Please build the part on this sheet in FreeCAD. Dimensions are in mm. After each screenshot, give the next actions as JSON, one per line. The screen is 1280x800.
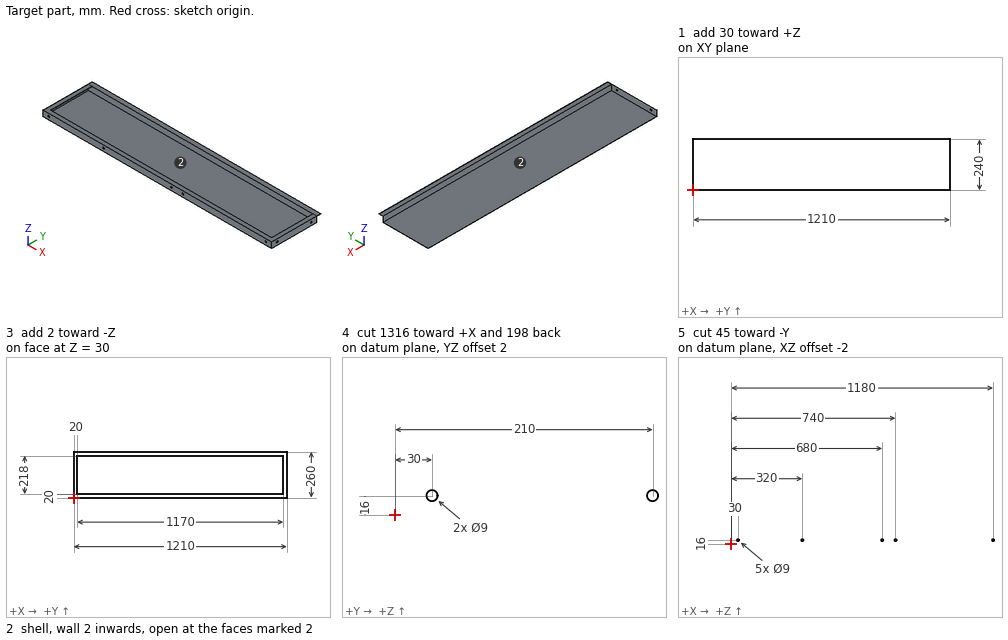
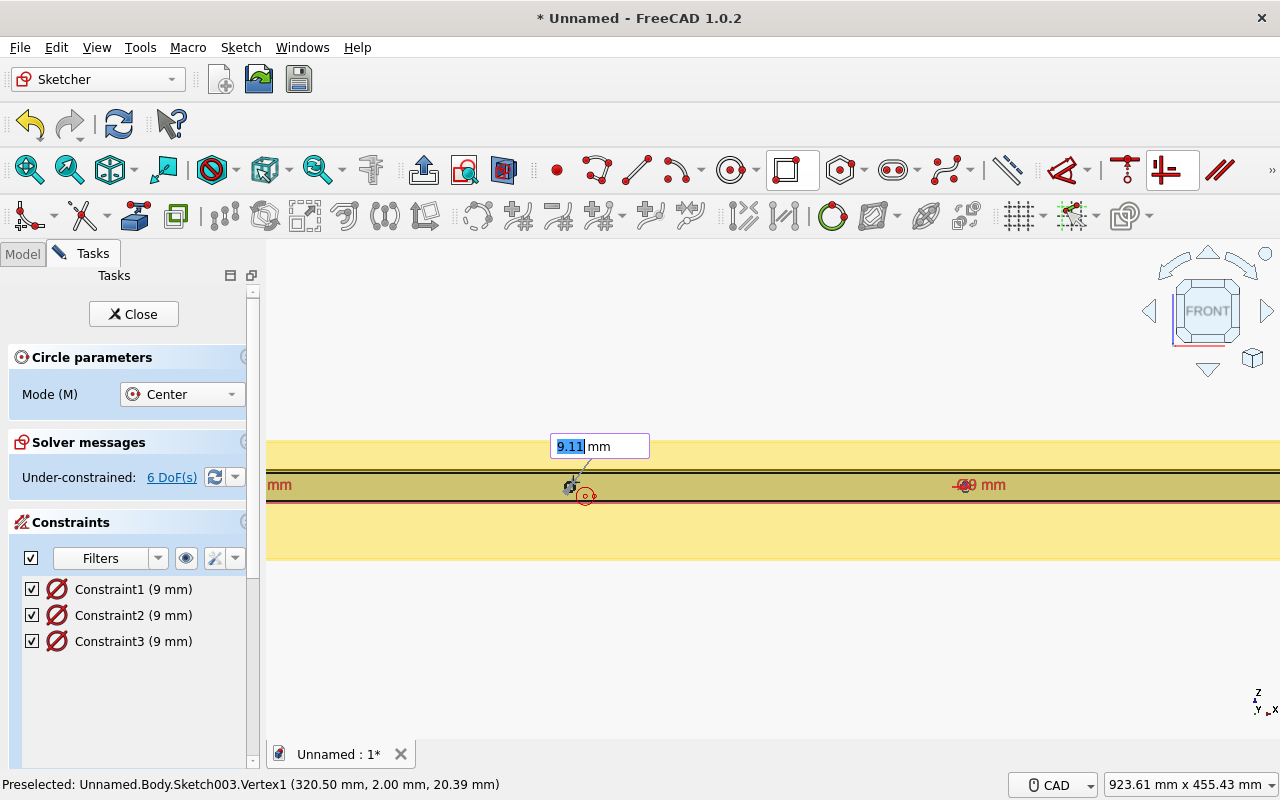
{"action": "type", "text": "9"}
{"action": "key", "text": "Return"}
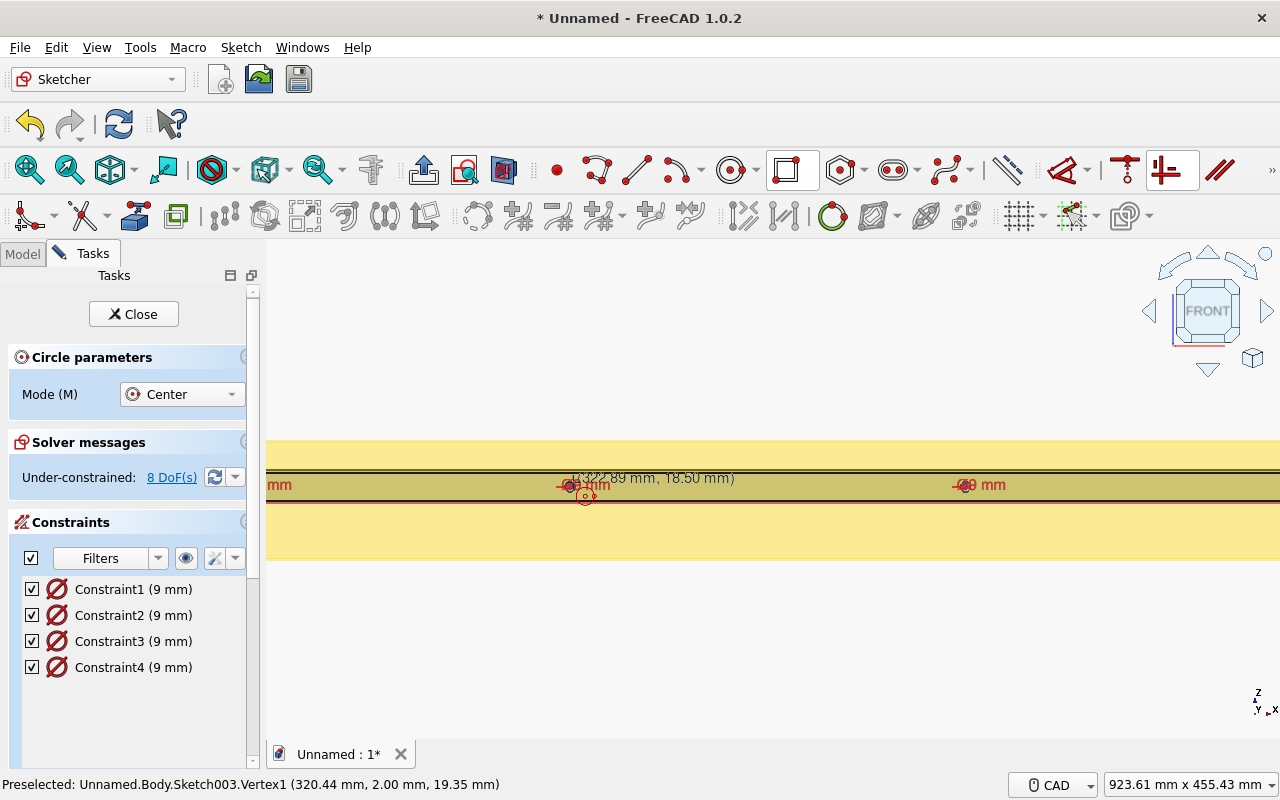
{"action": "scroll", "coordinate": [1031, 486], "scroll_direction": "up", "scroll_amount": 8}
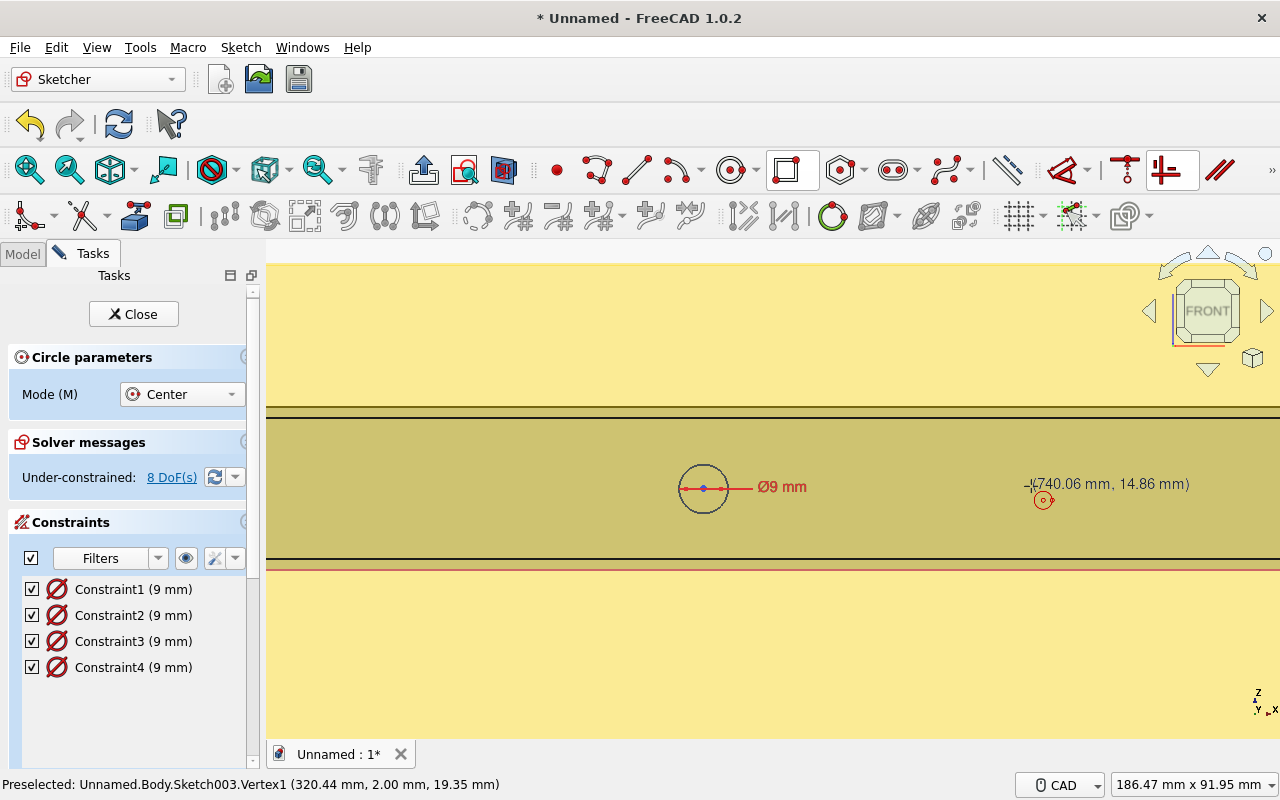
{"action": "scroll", "coordinate": [752, 486], "scroll_direction": "down", "scroll_amount": 12}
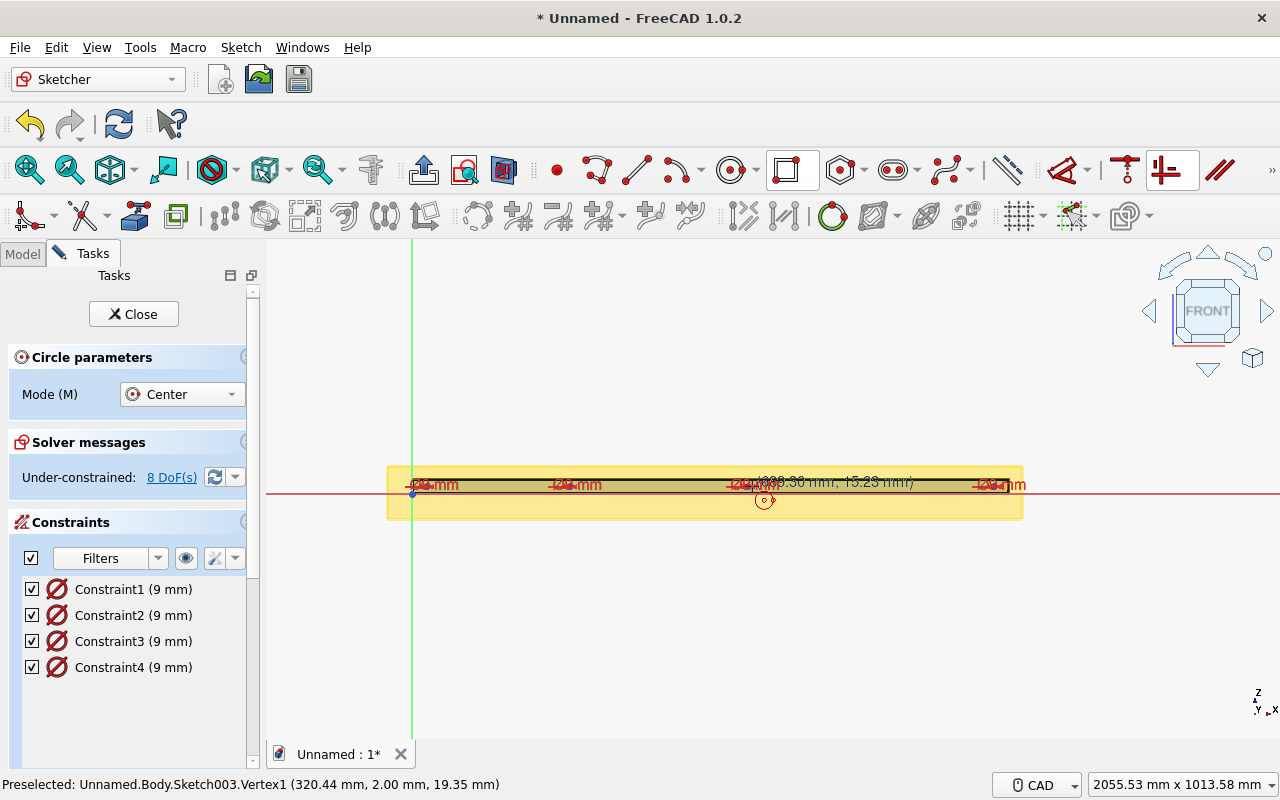
{"action": "scroll", "coordinate": [777, 486], "scroll_direction": "up", "scroll_amount": 4}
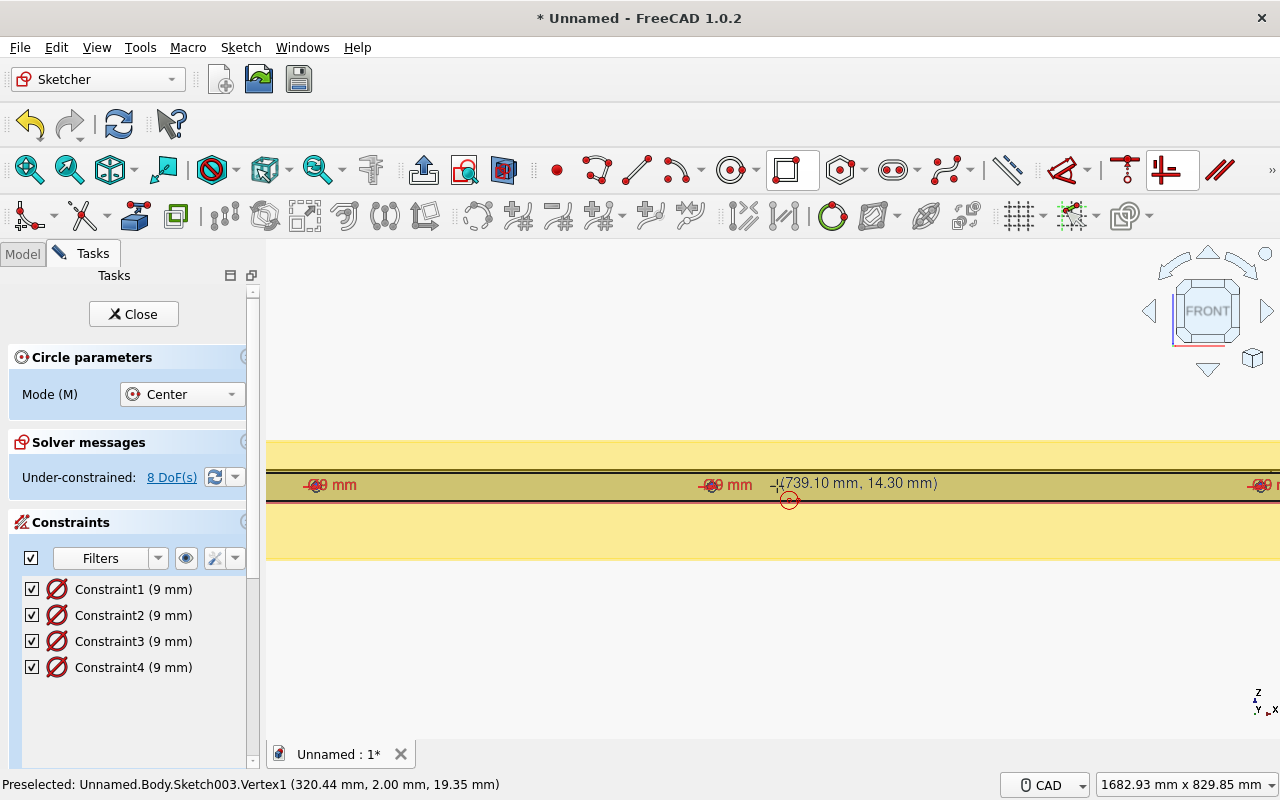
{"action": "left_click", "coordinate": [777, 486]}
{"action": "mouse_move", "coordinate": [781, 482]}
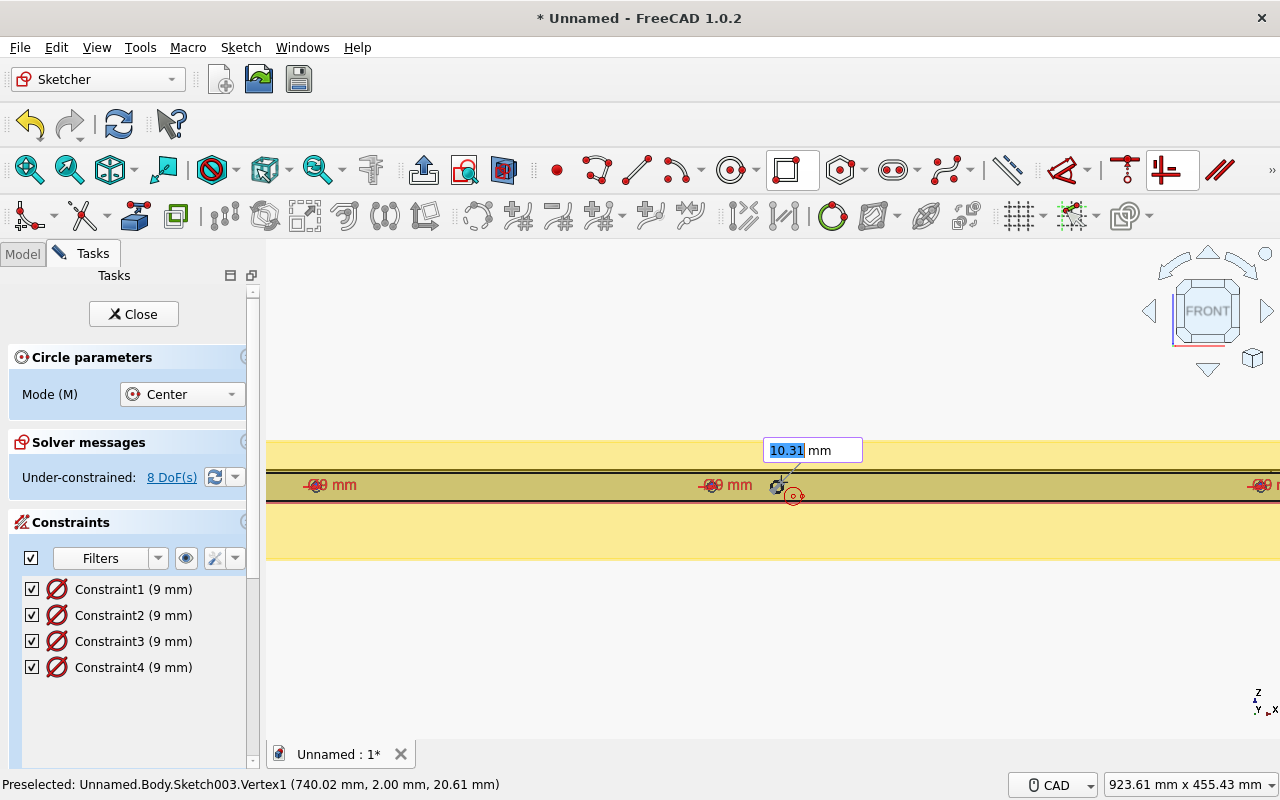
{"action": "type", "text": "9"}
{"action": "key", "text": "Return"}
{"action": "key", "text": "Escape"}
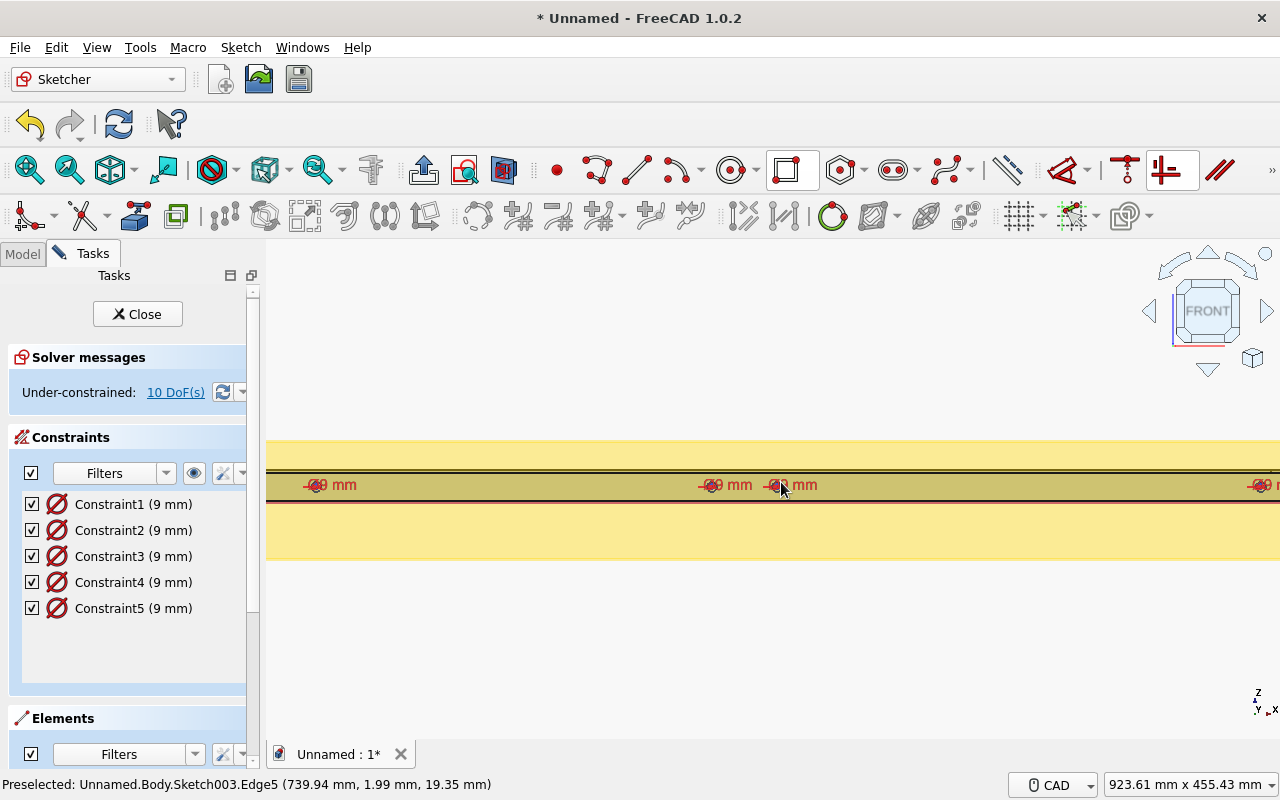
{"action": "scroll", "coordinate": [777, 487], "scroll_direction": "down", "scroll_amount": 4}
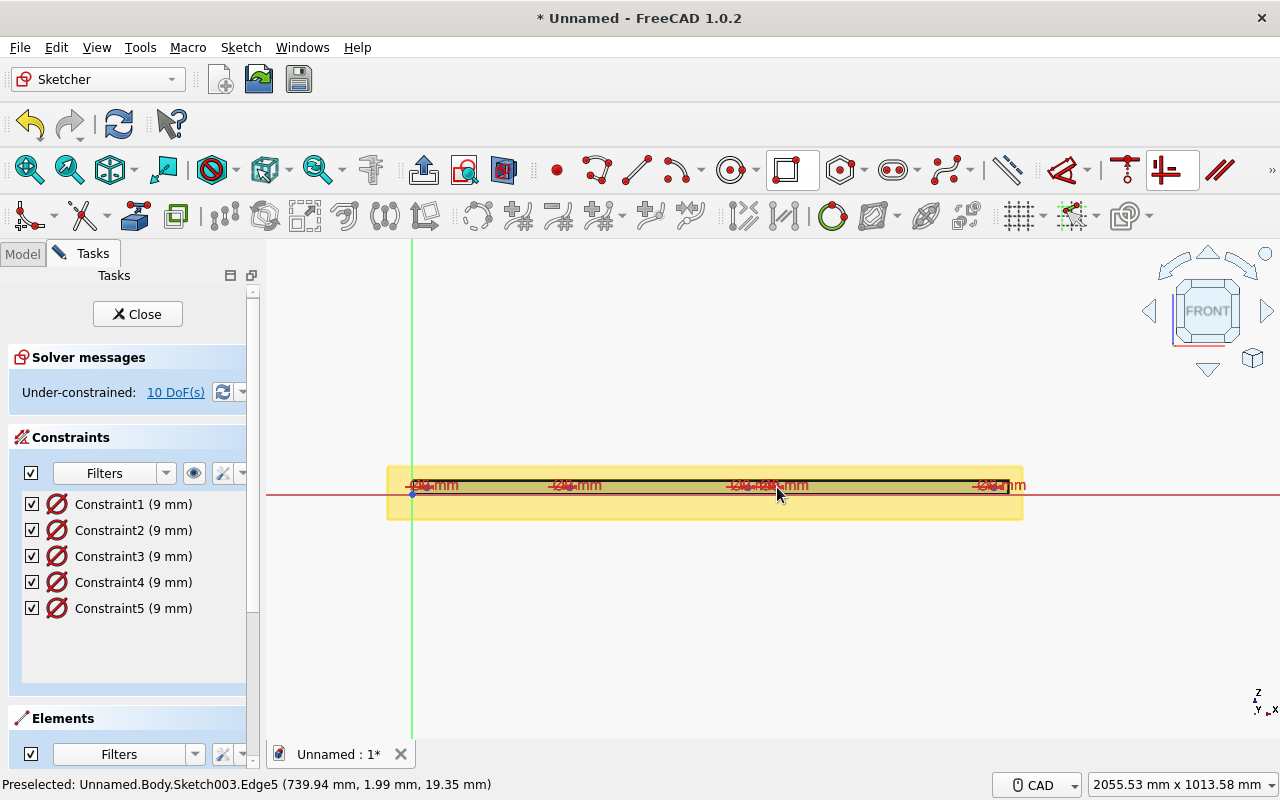
{"action": "left_click", "coordinate": [427, 487]}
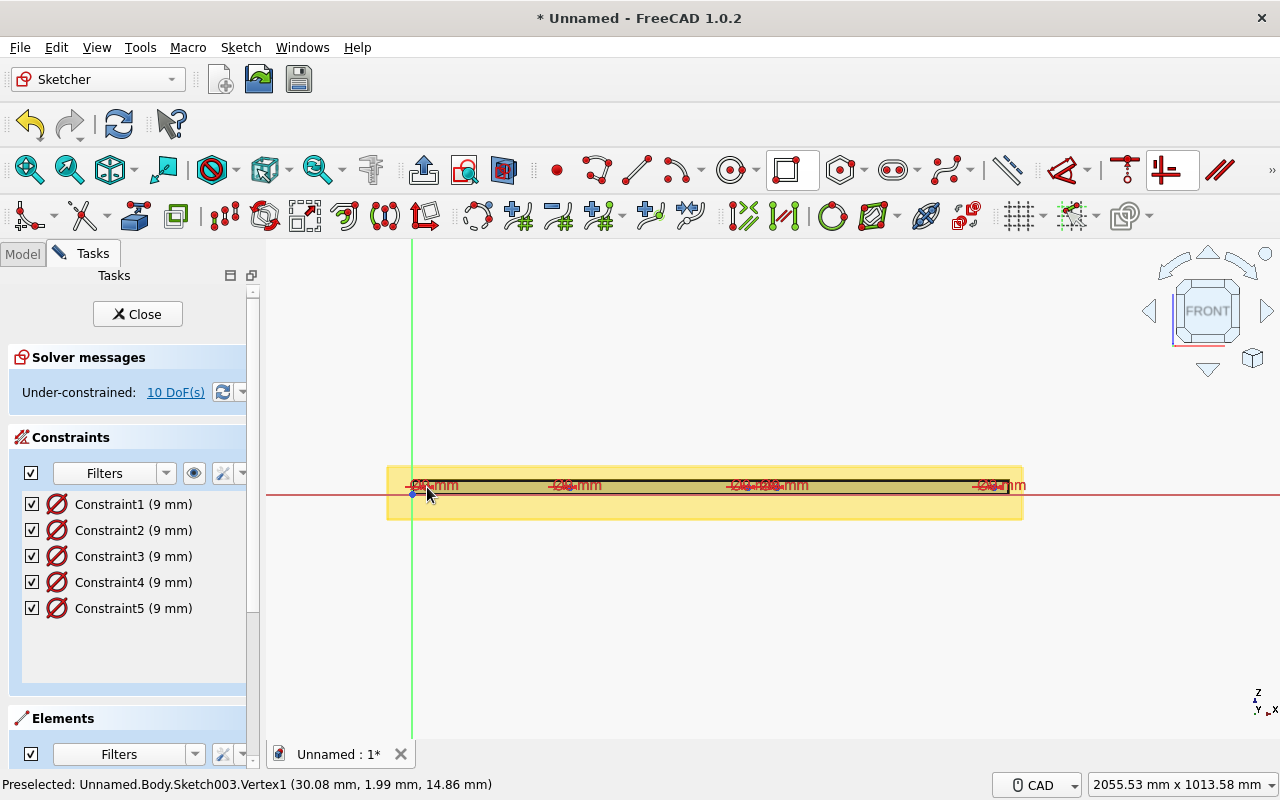
{"action": "left_click", "coordinate": [995, 487]}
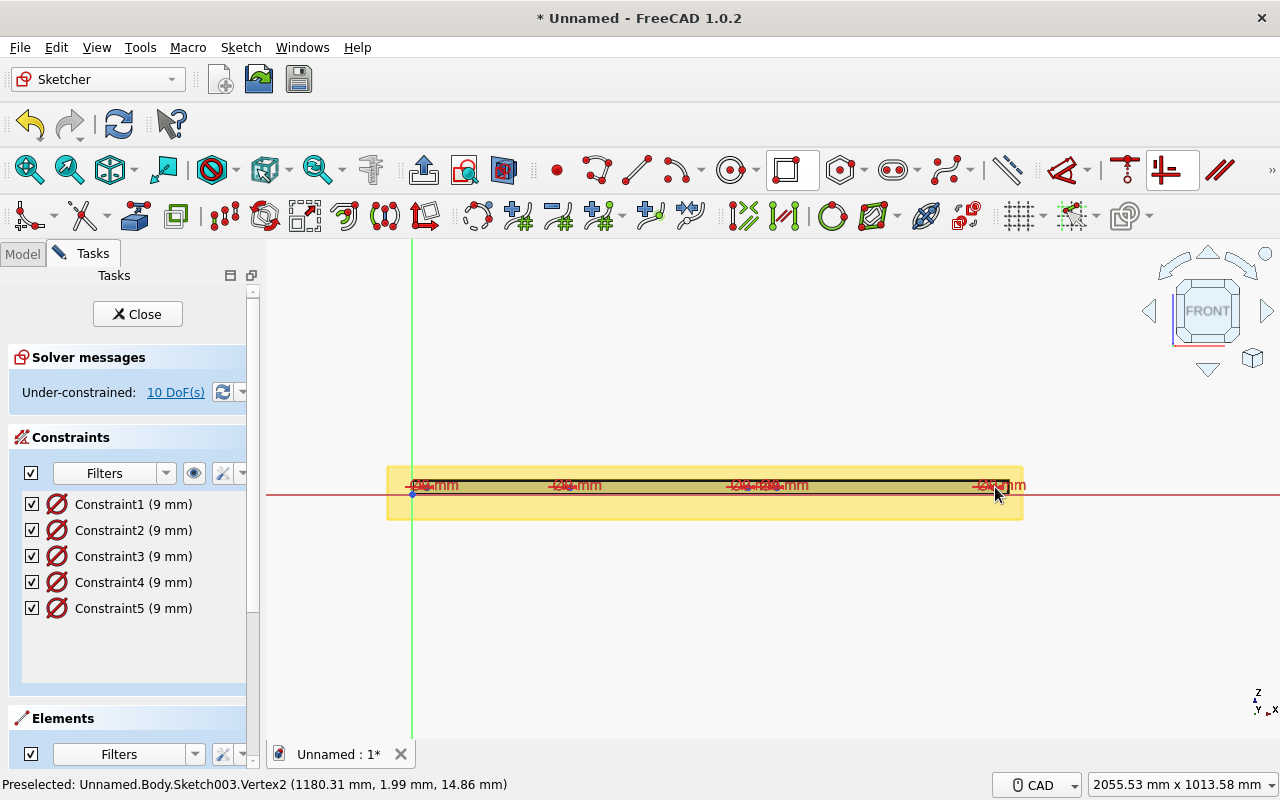
{"action": "left_click", "coordinate": [1194, 170]}